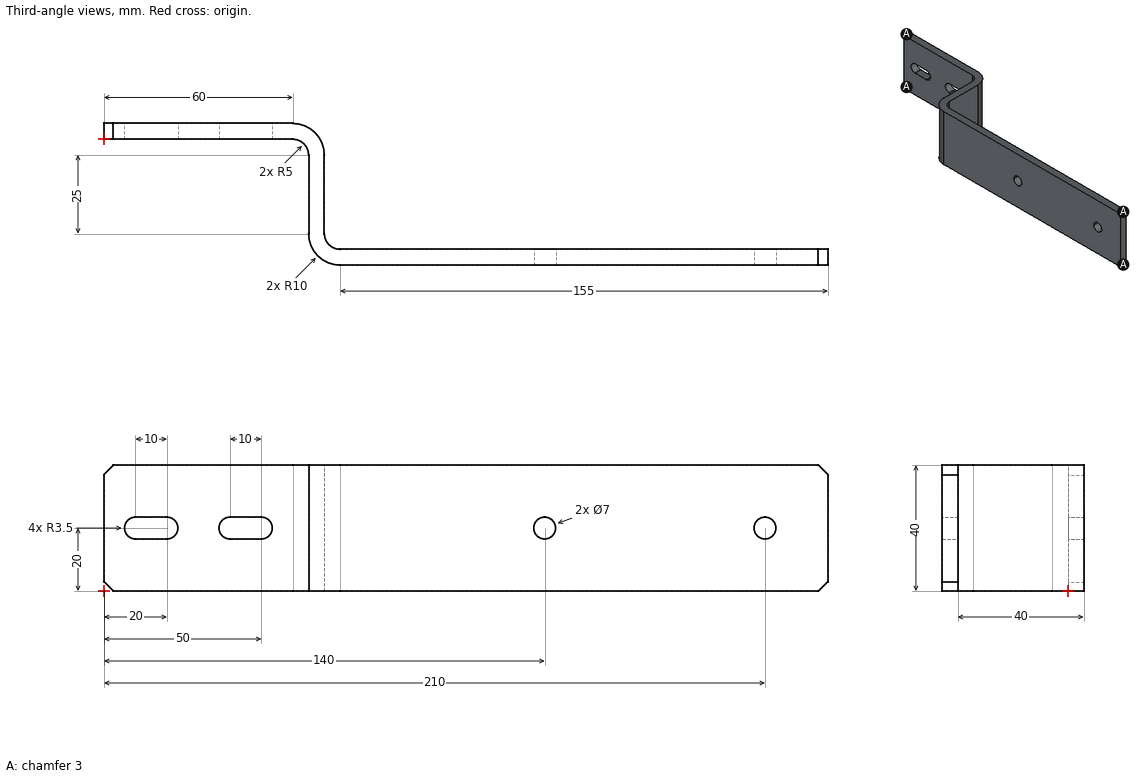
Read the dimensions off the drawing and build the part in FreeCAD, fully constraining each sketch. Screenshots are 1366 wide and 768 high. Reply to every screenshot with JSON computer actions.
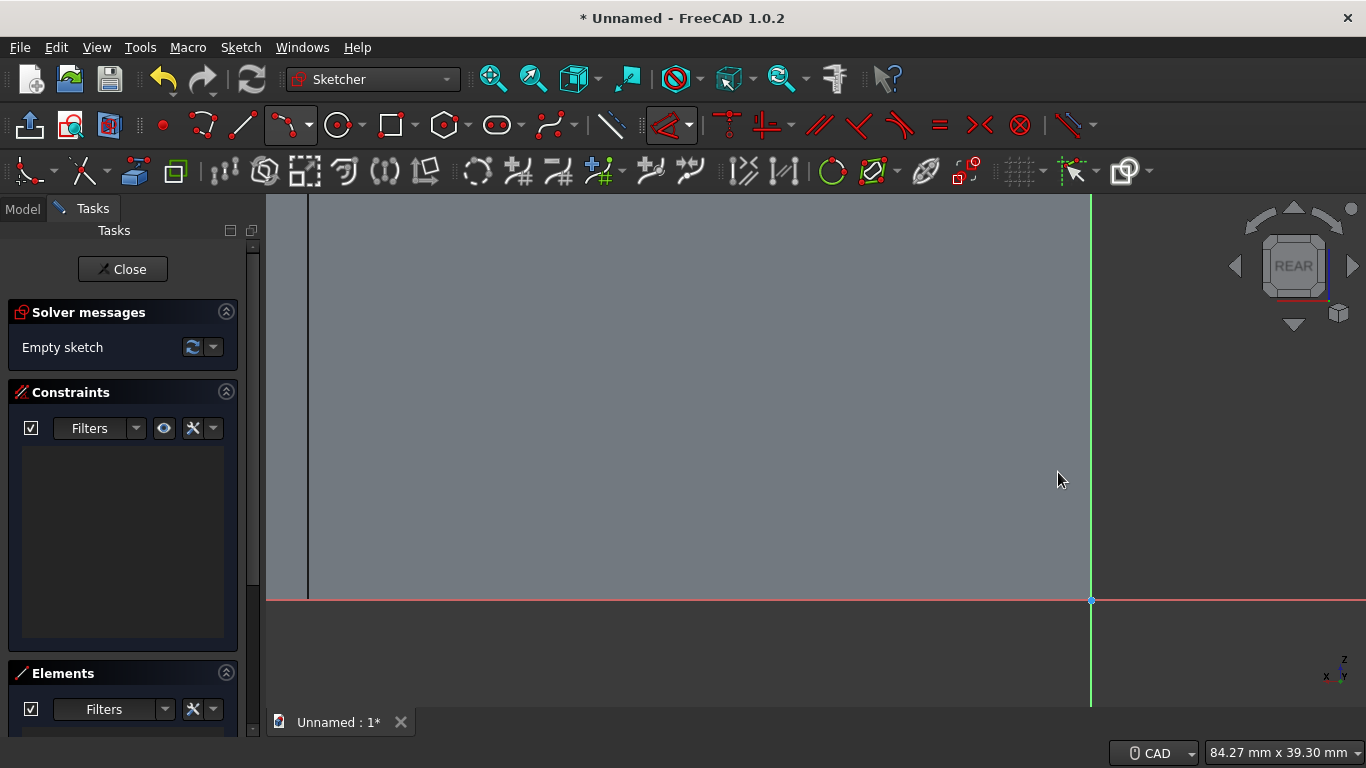
{"action": "left_click", "coordinate": [498, 126]}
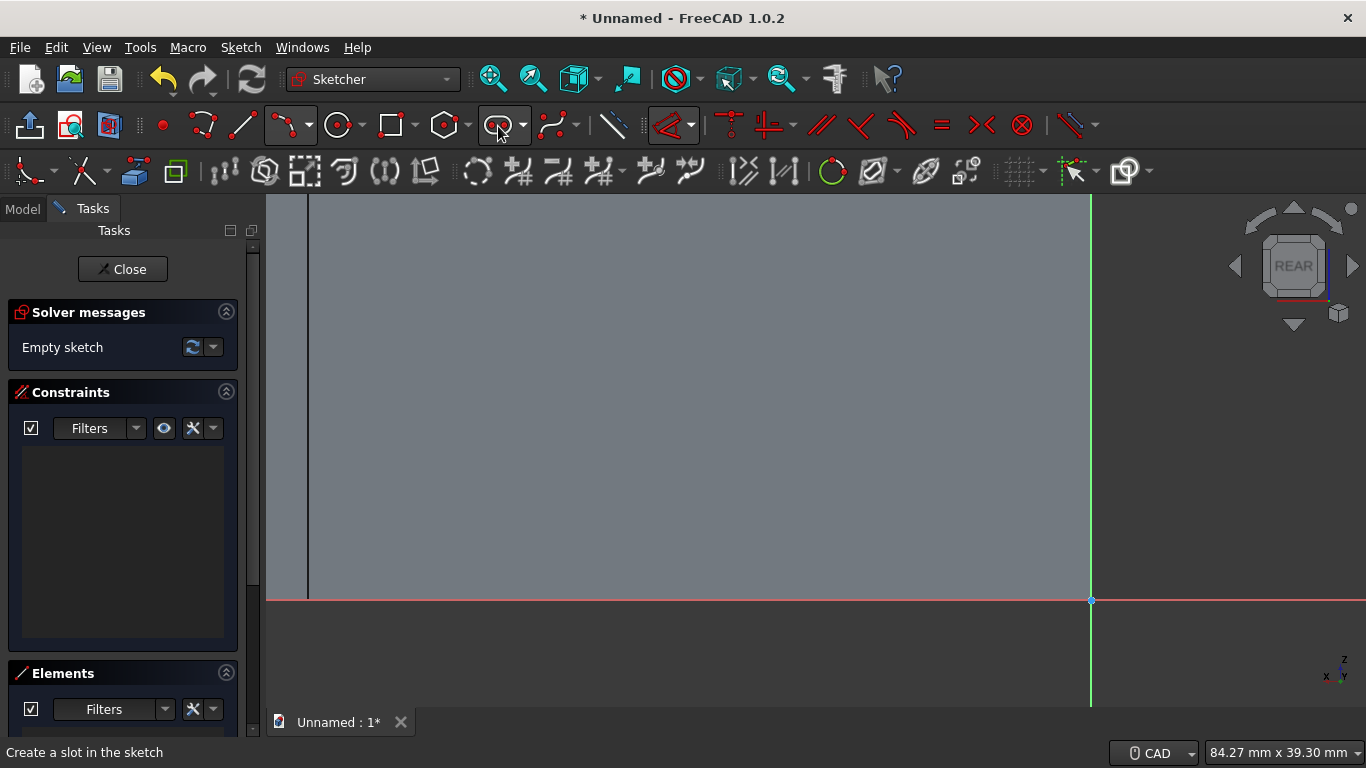
{"action": "left_click", "coordinate": [830, 339]}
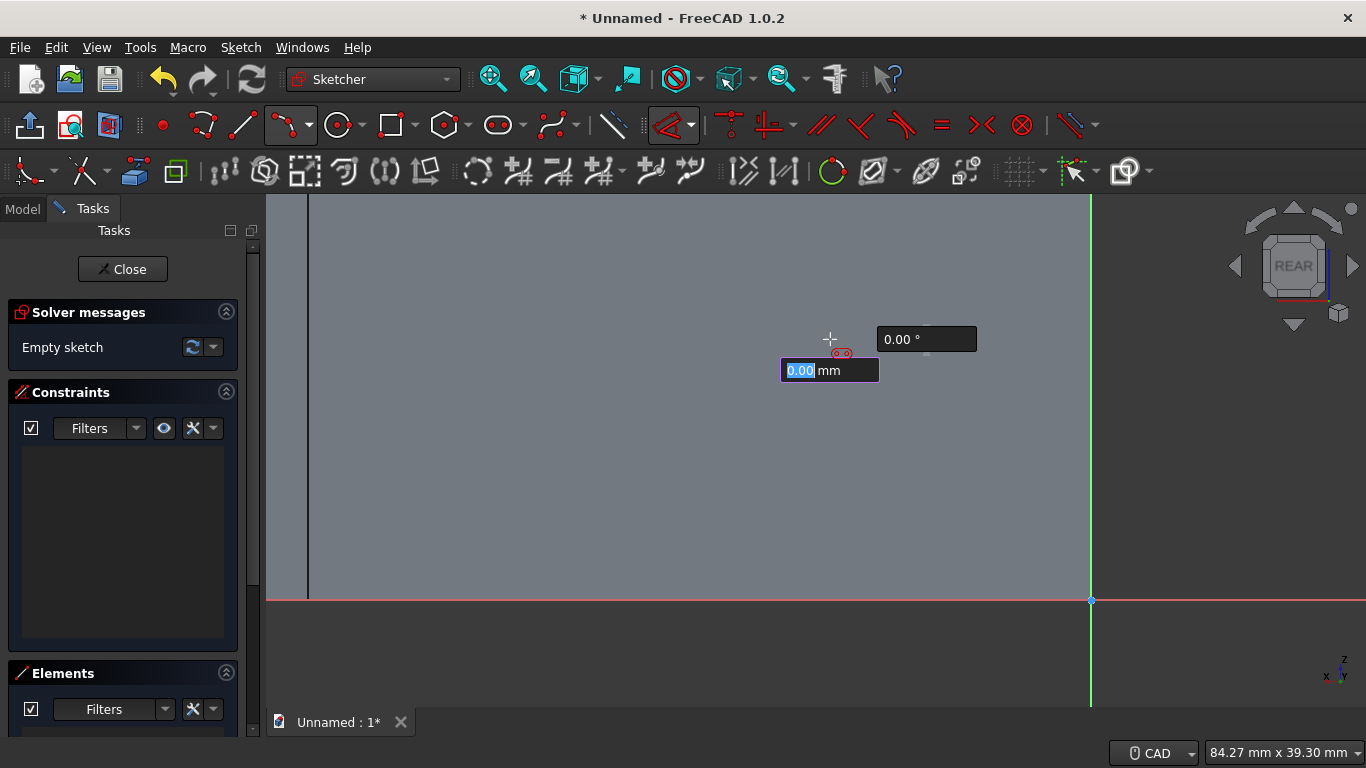
{"action": "left_click", "coordinate": [961, 339]}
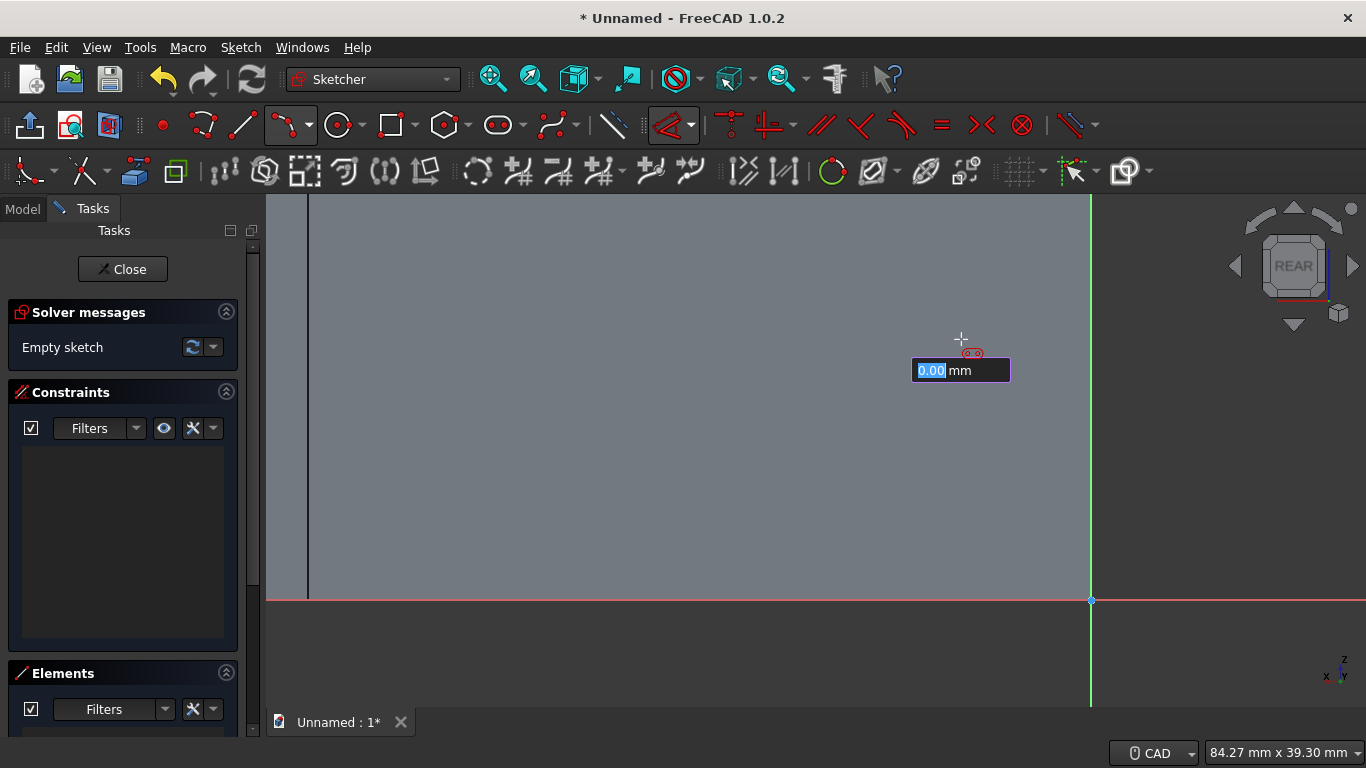
{"action": "left_click", "coordinate": [896, 385]}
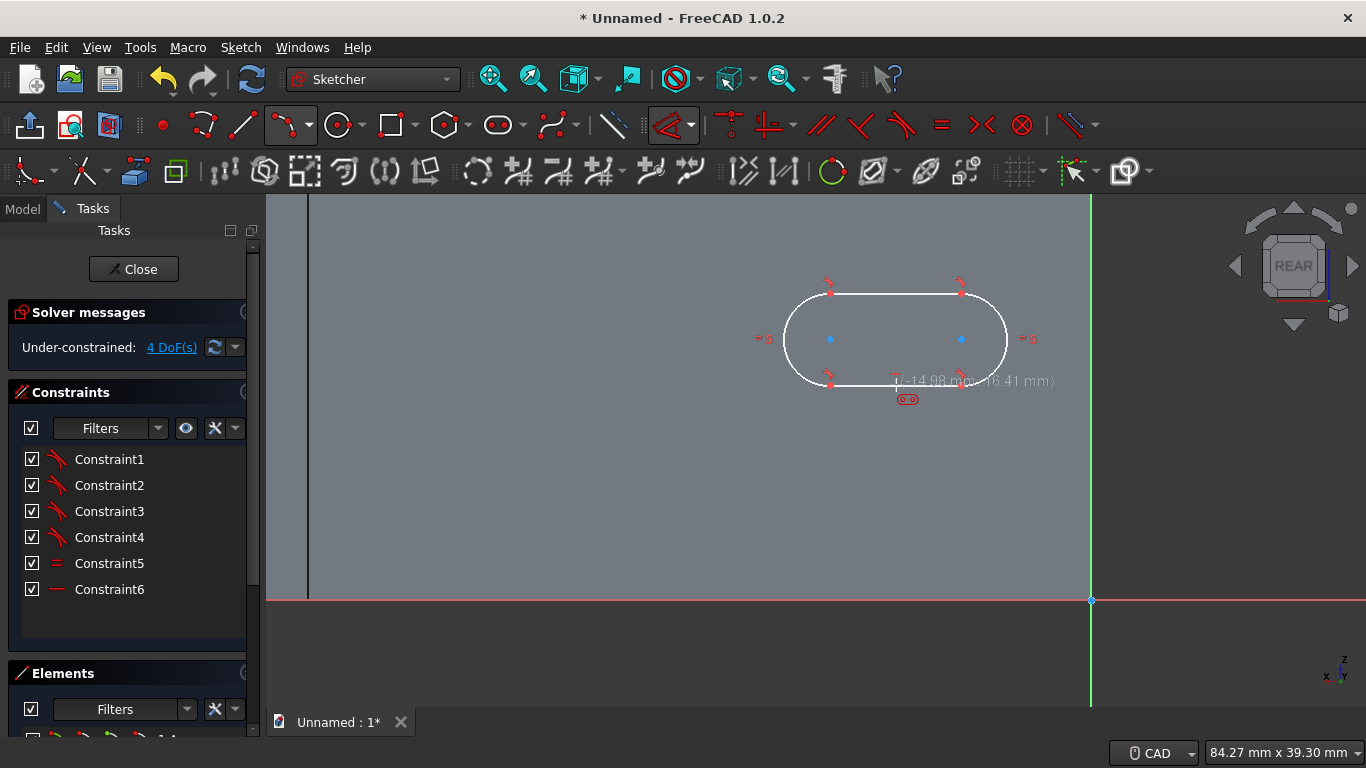
{"action": "left_click", "coordinate": [439, 339]}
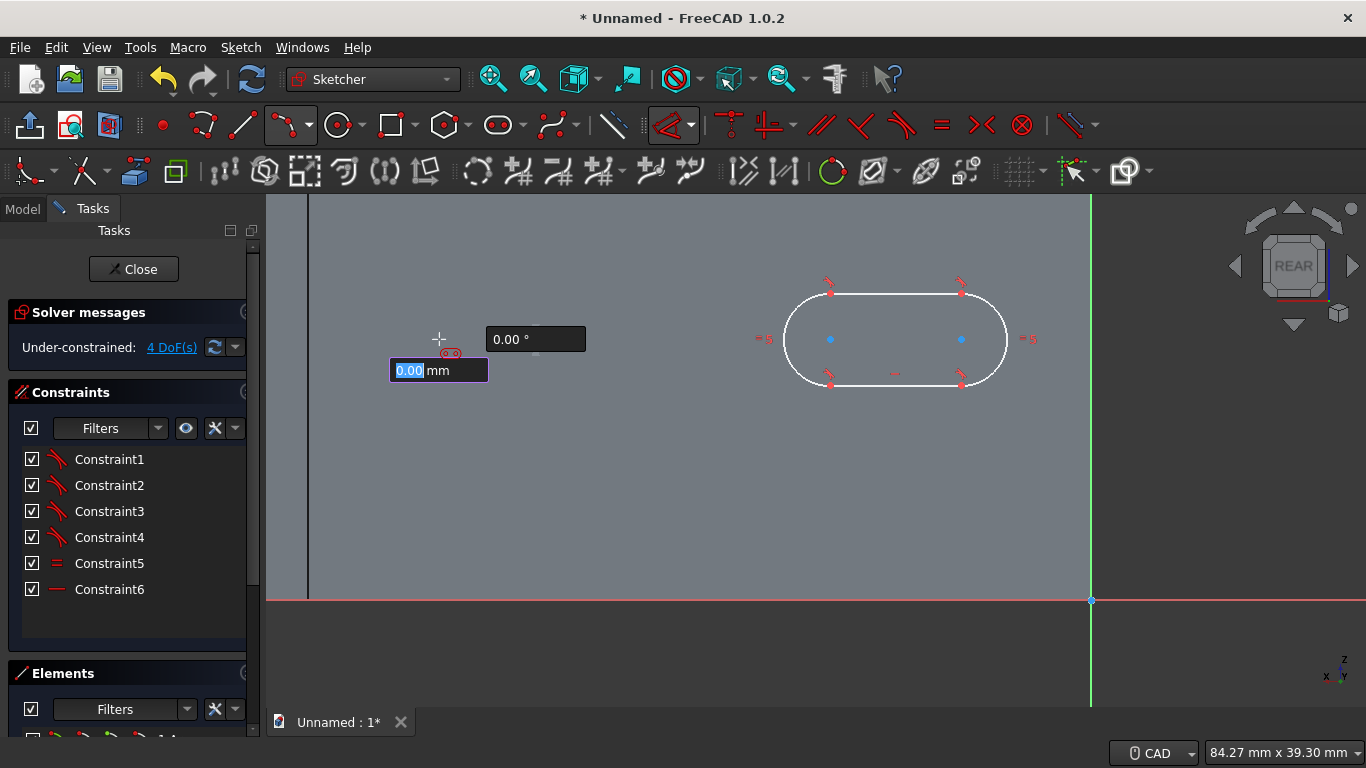
{"action": "left_click", "coordinate": [569, 339]}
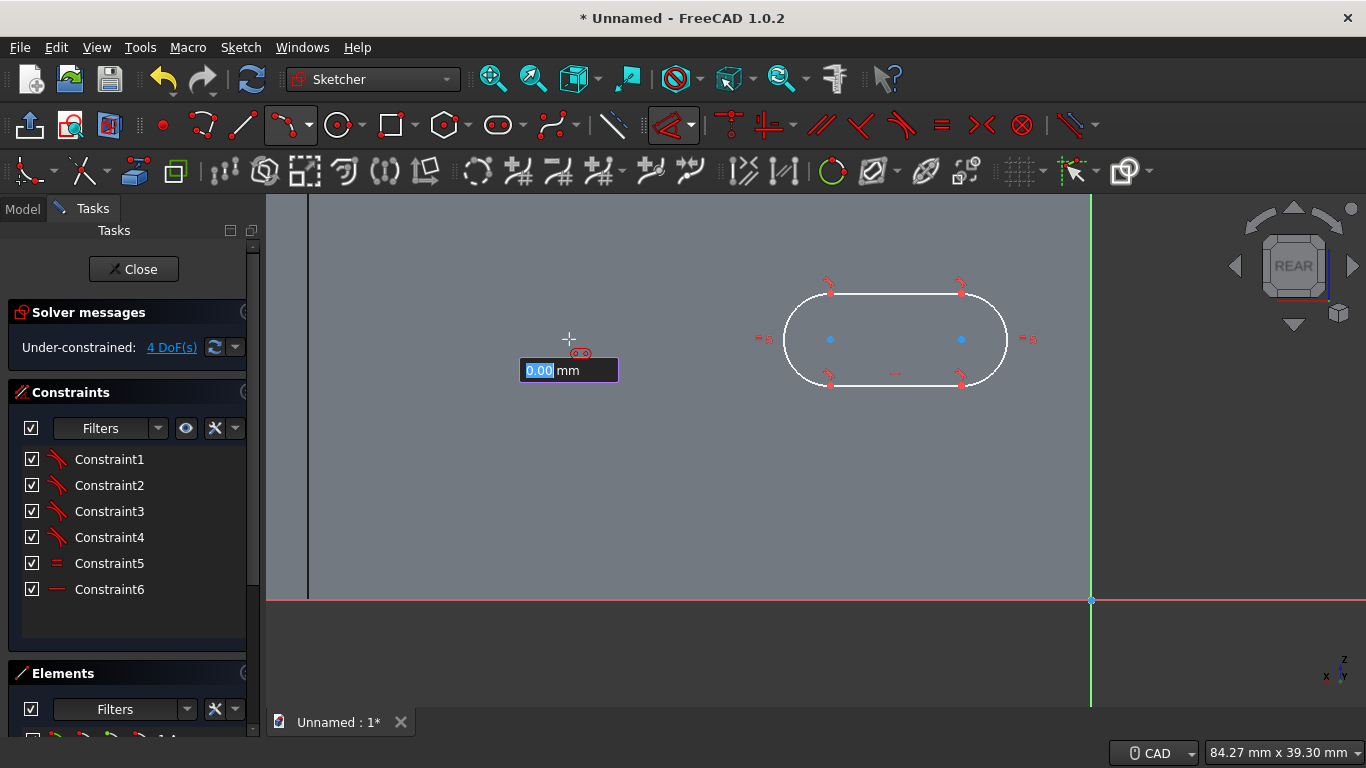
{"action": "left_click", "coordinate": [504, 385]}
{"action": "key", "text": "Escape"}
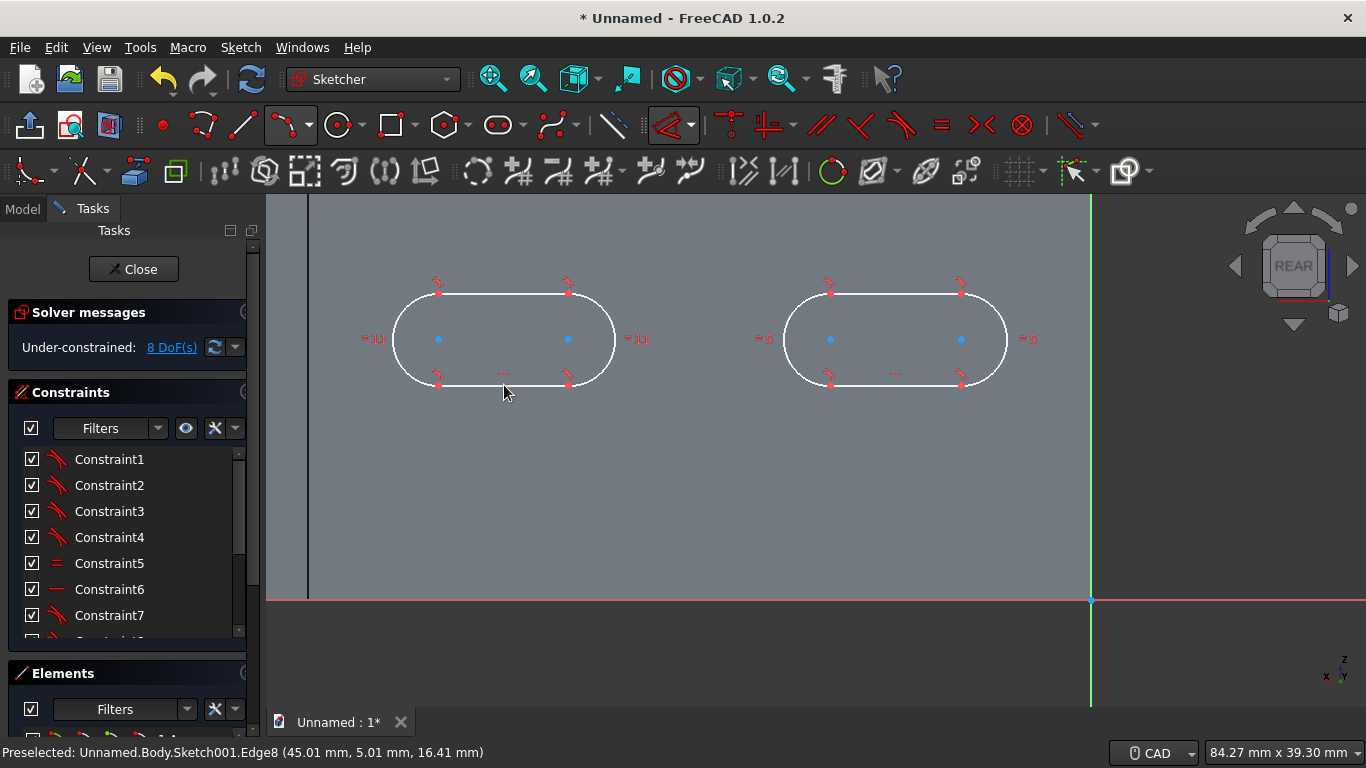
{"action": "left_click", "coordinate": [793, 313]}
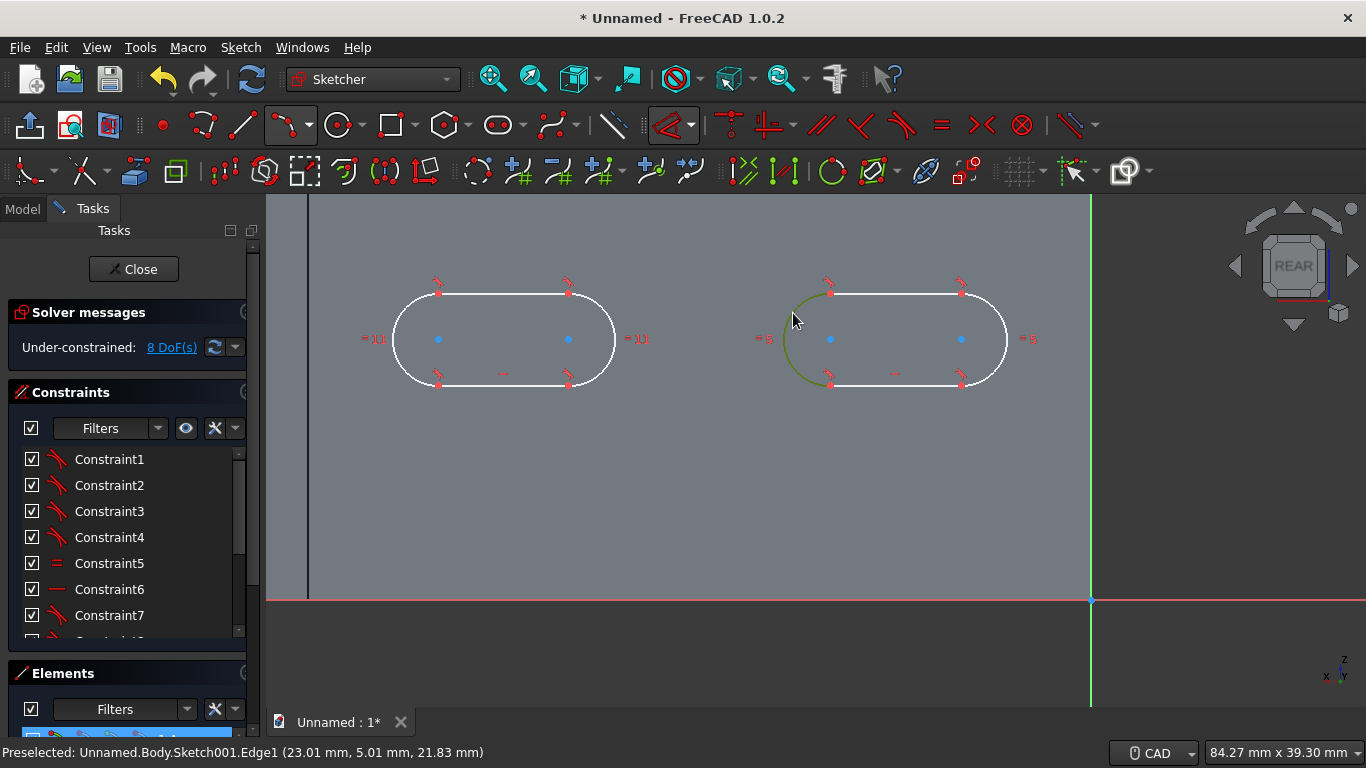
{"action": "left_click", "coordinate": [402, 313]}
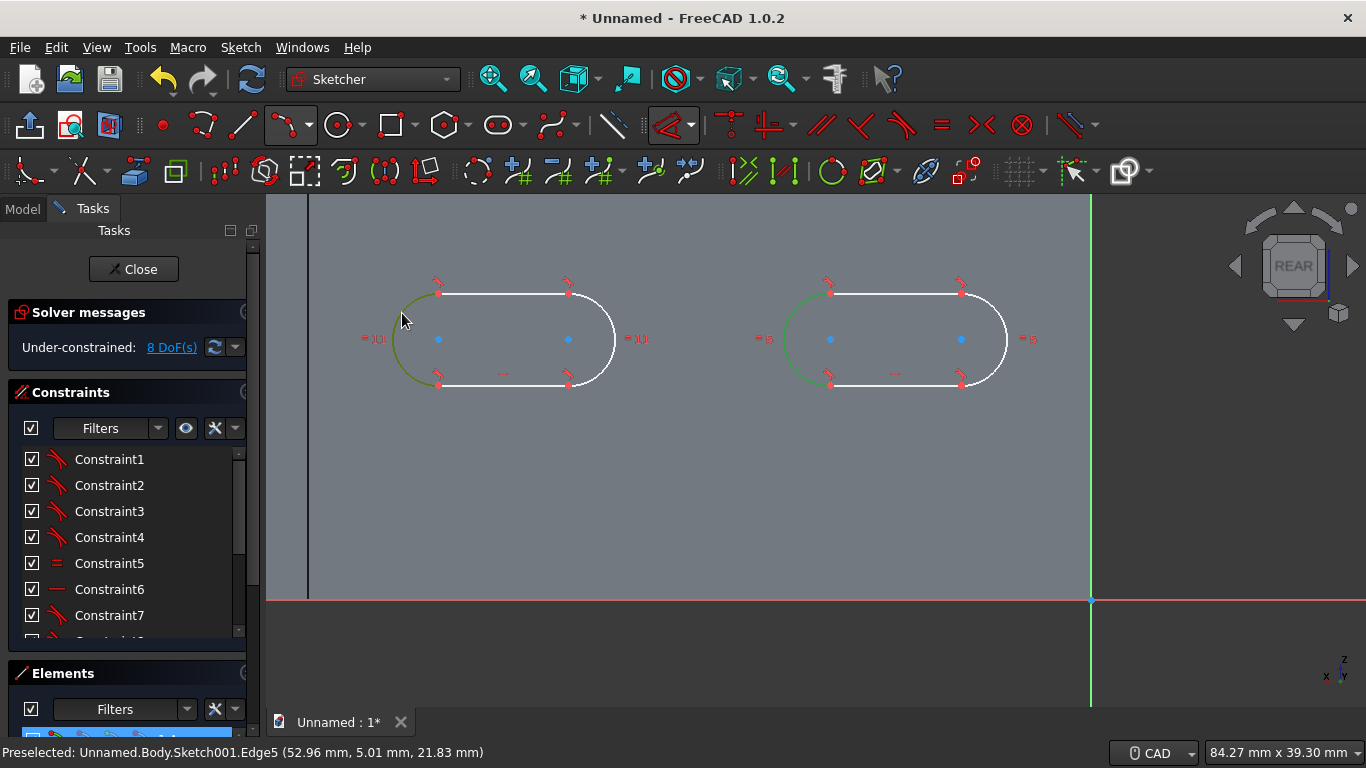
{"action": "left_click", "coordinate": [942, 126]}